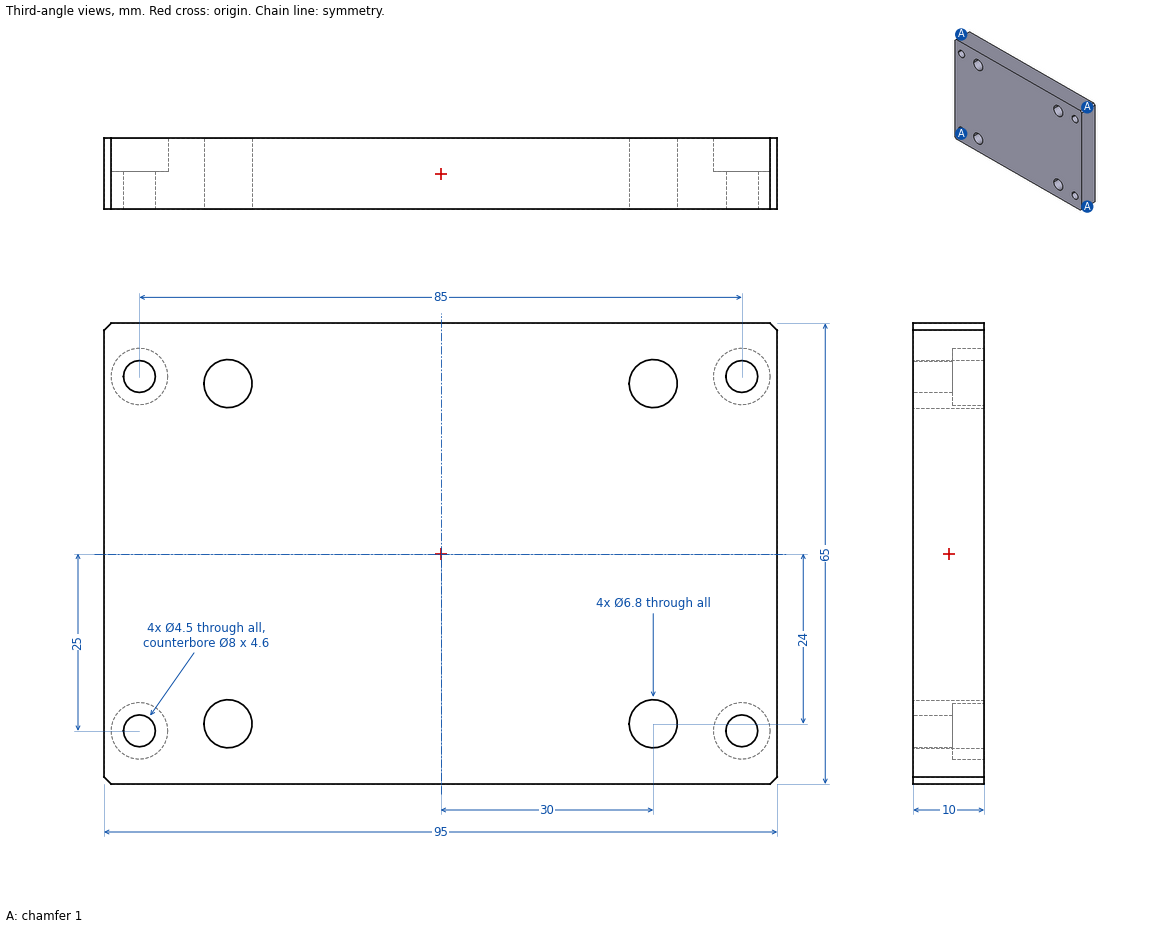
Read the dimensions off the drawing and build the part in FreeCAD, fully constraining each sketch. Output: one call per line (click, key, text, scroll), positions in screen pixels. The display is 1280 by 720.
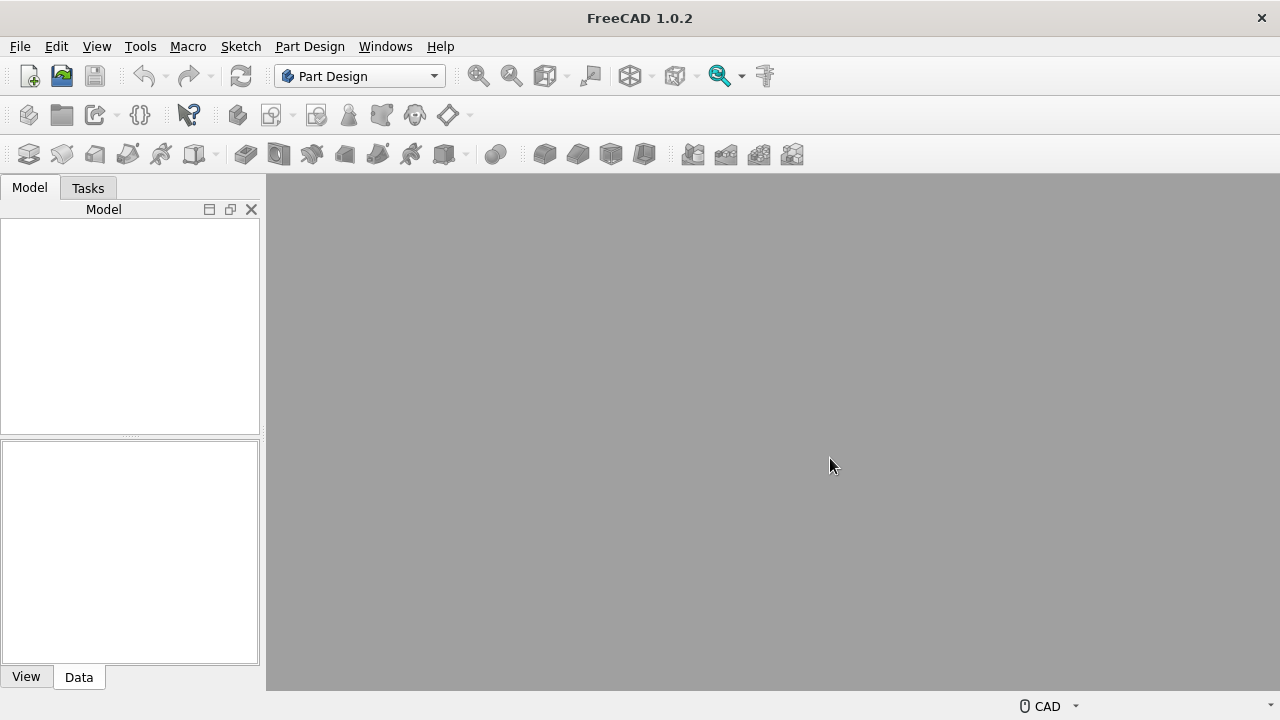
key(ctrl+n)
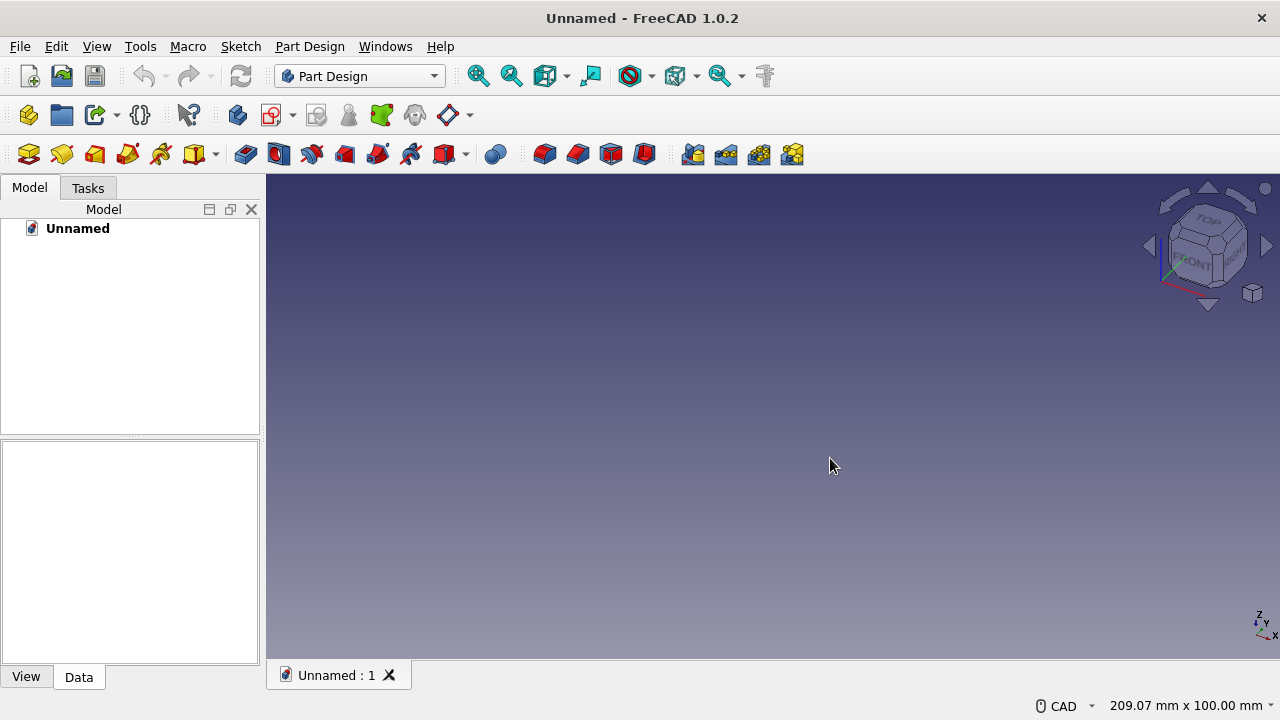
click(270, 116)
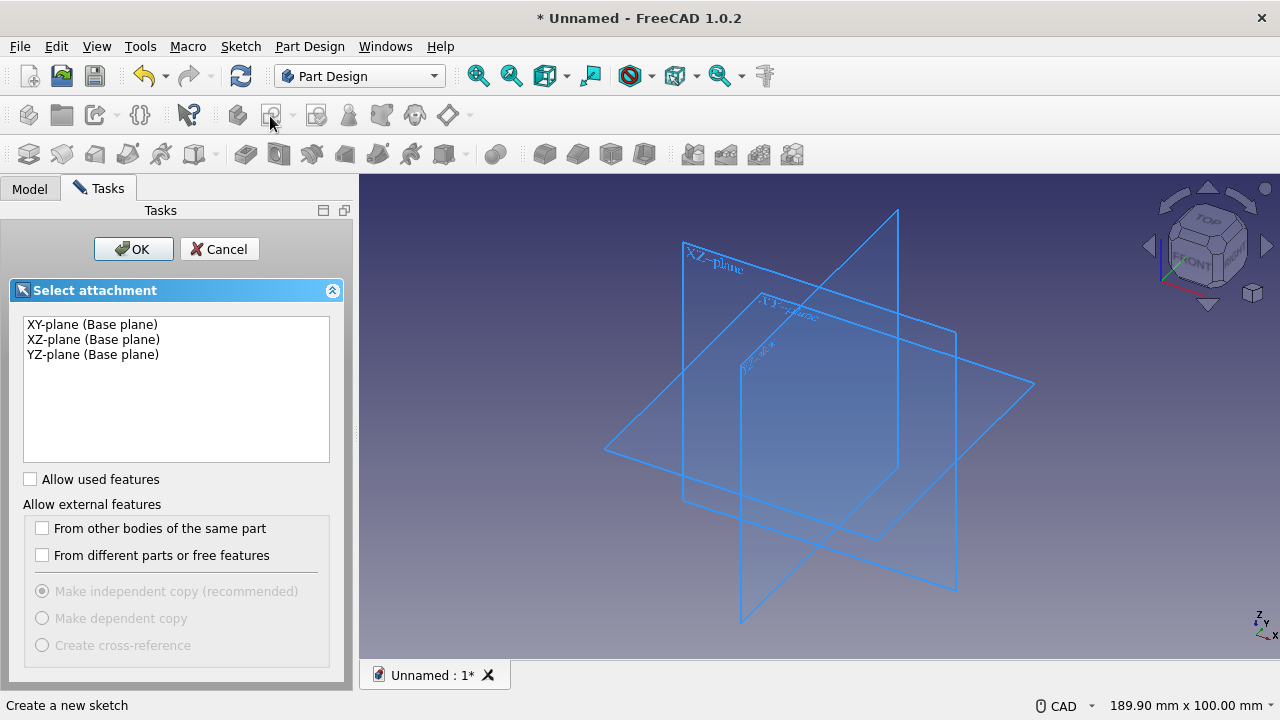
click(84, 340)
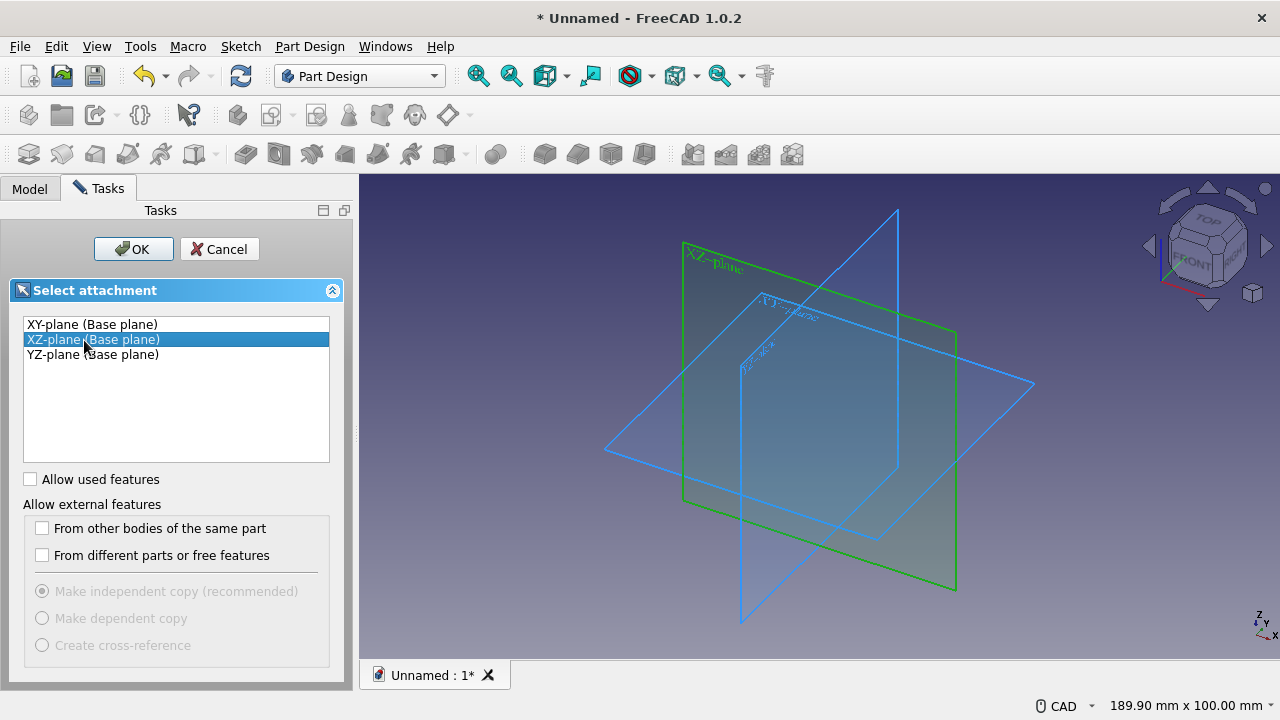
click(134, 249)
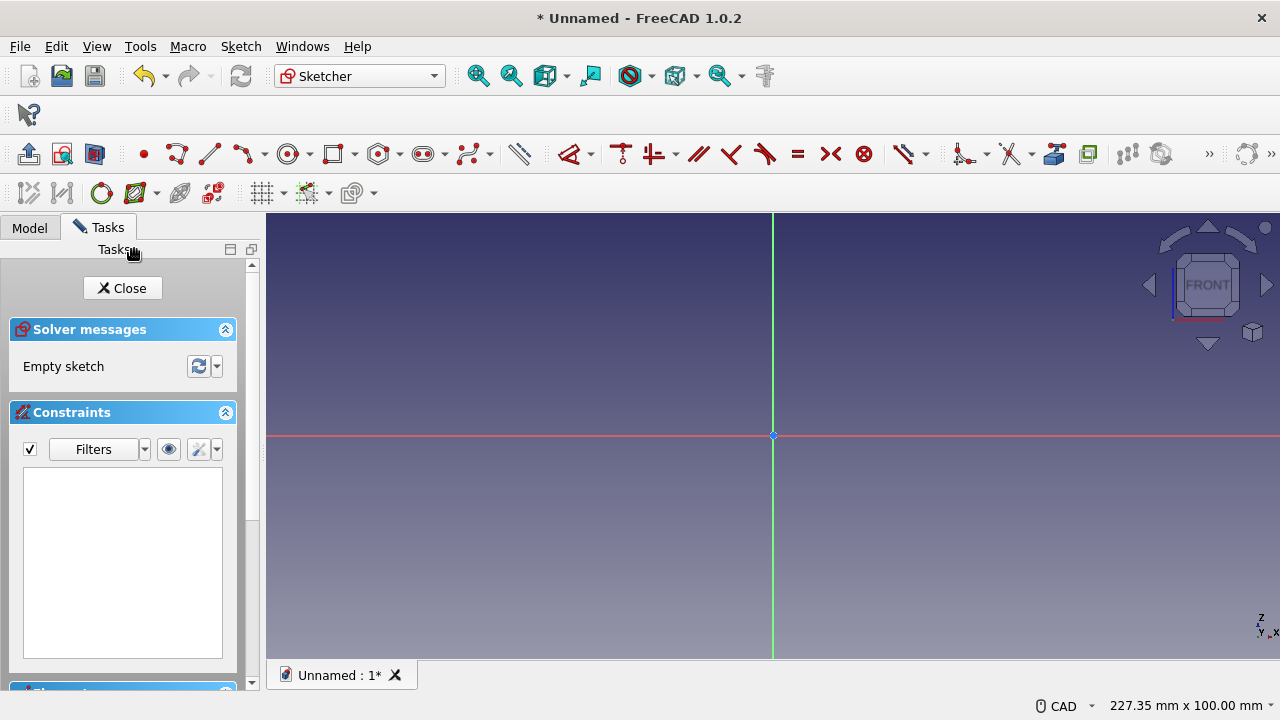
click(354, 154)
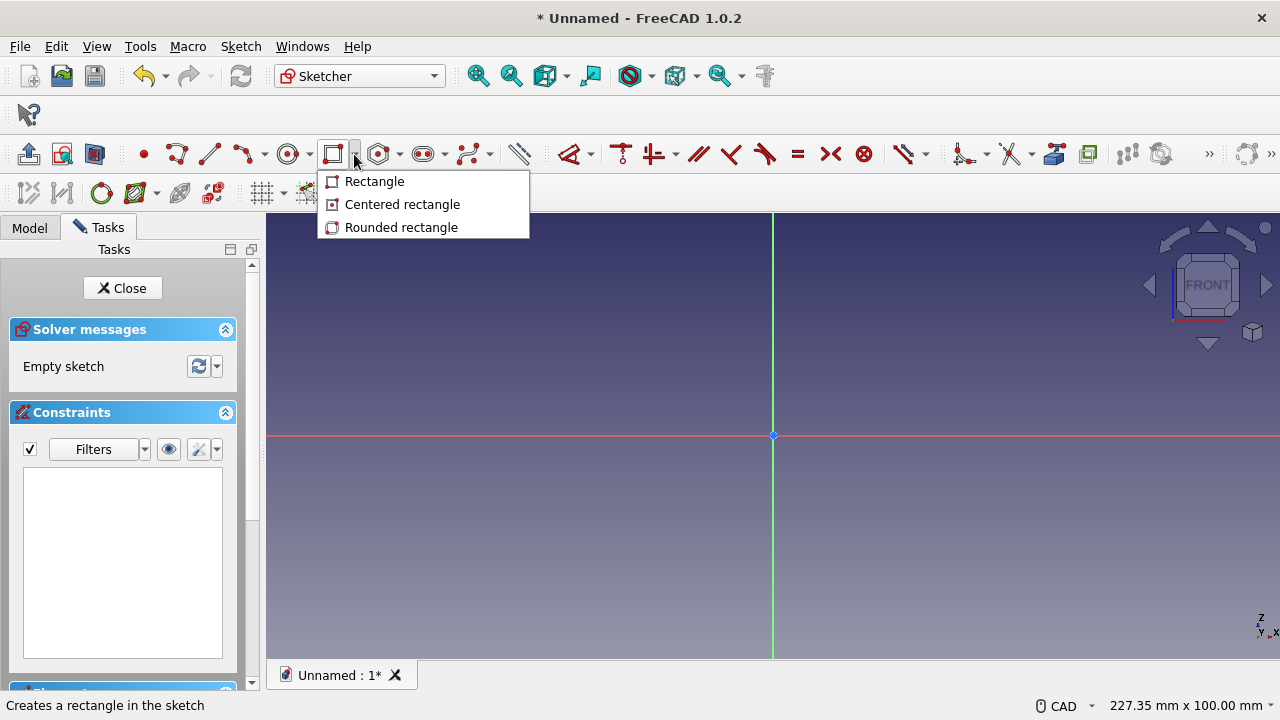
click(424, 204)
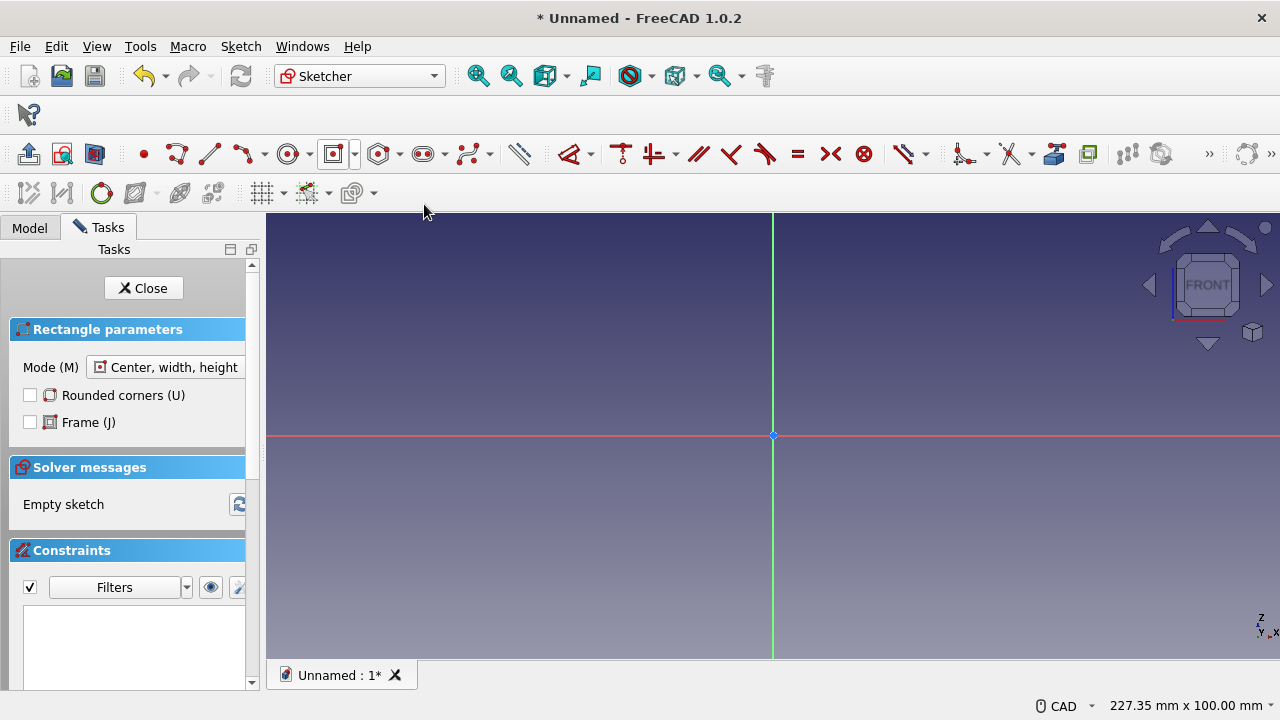
click(773, 436)
move(985, 291)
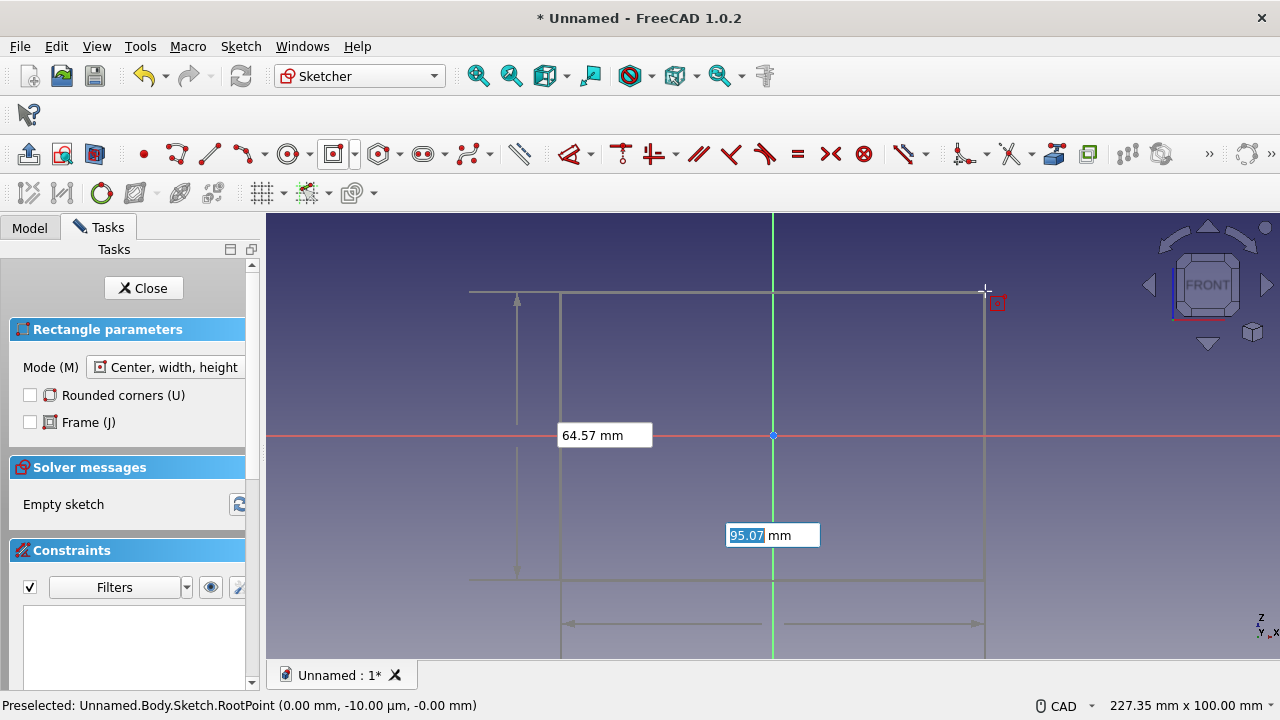
text(95)
key(Tab)
text(65)
key(Return)
key(Escape)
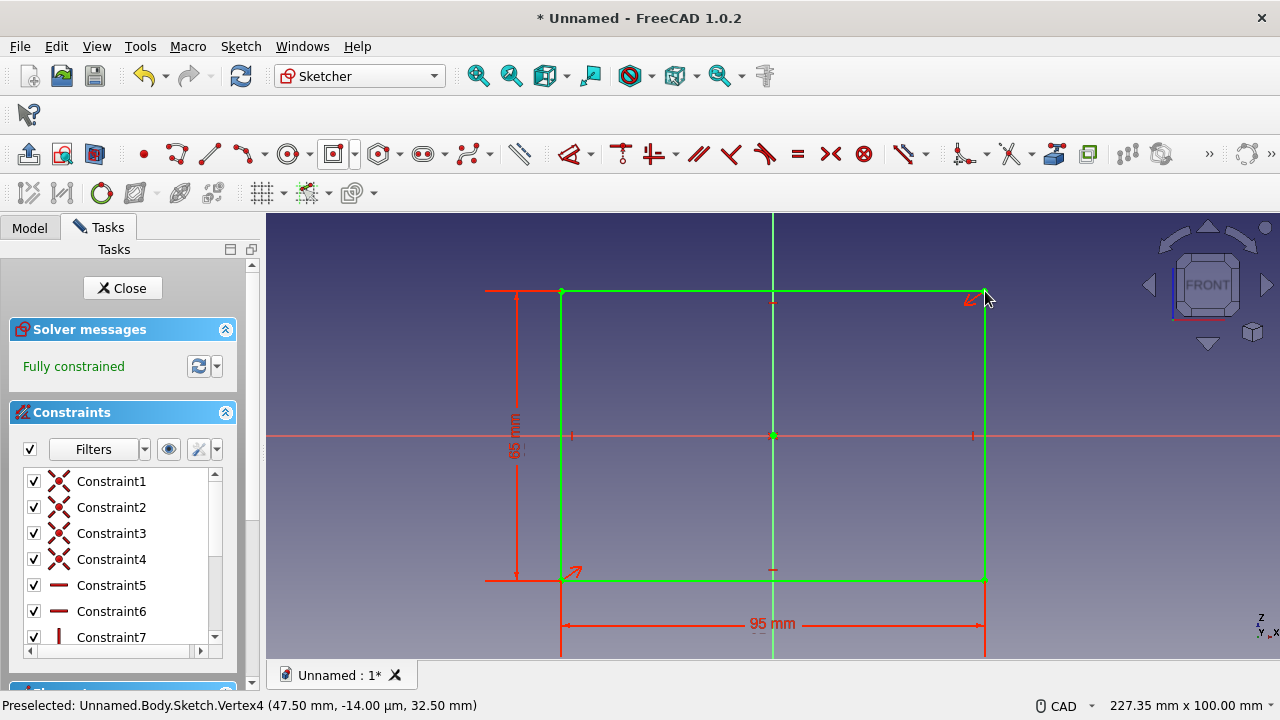
click(123, 288)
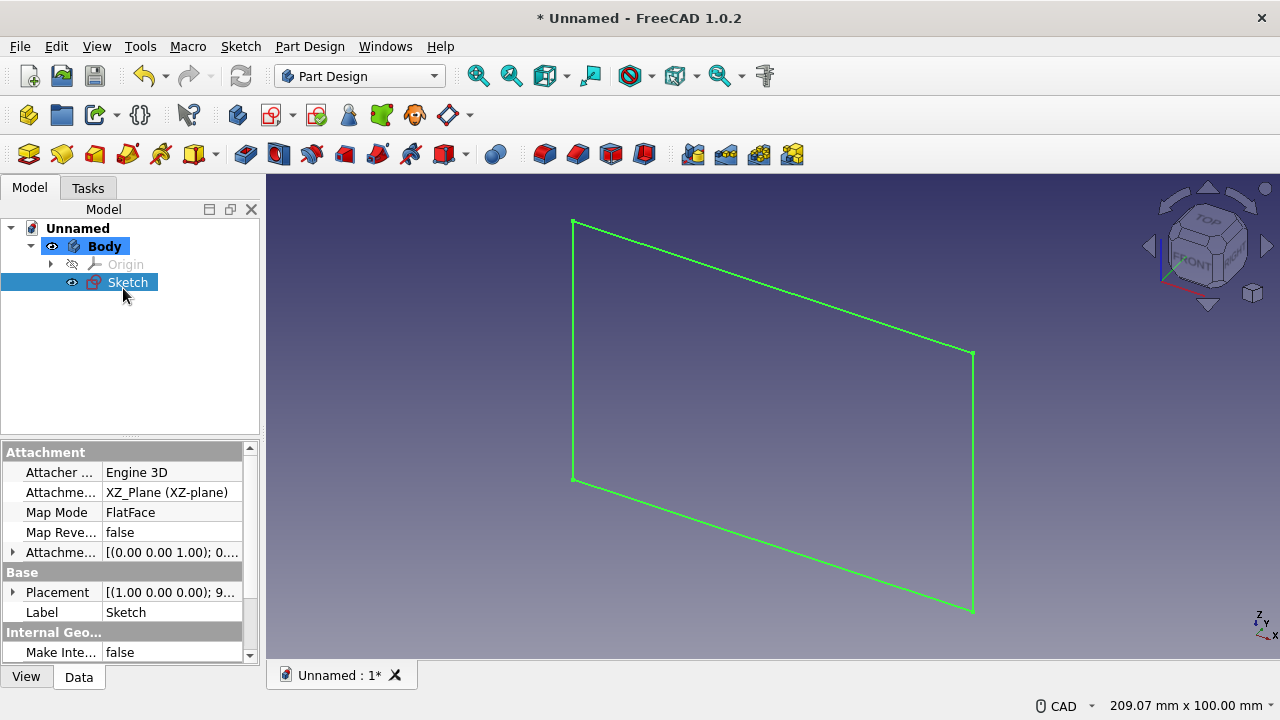
click(29, 154)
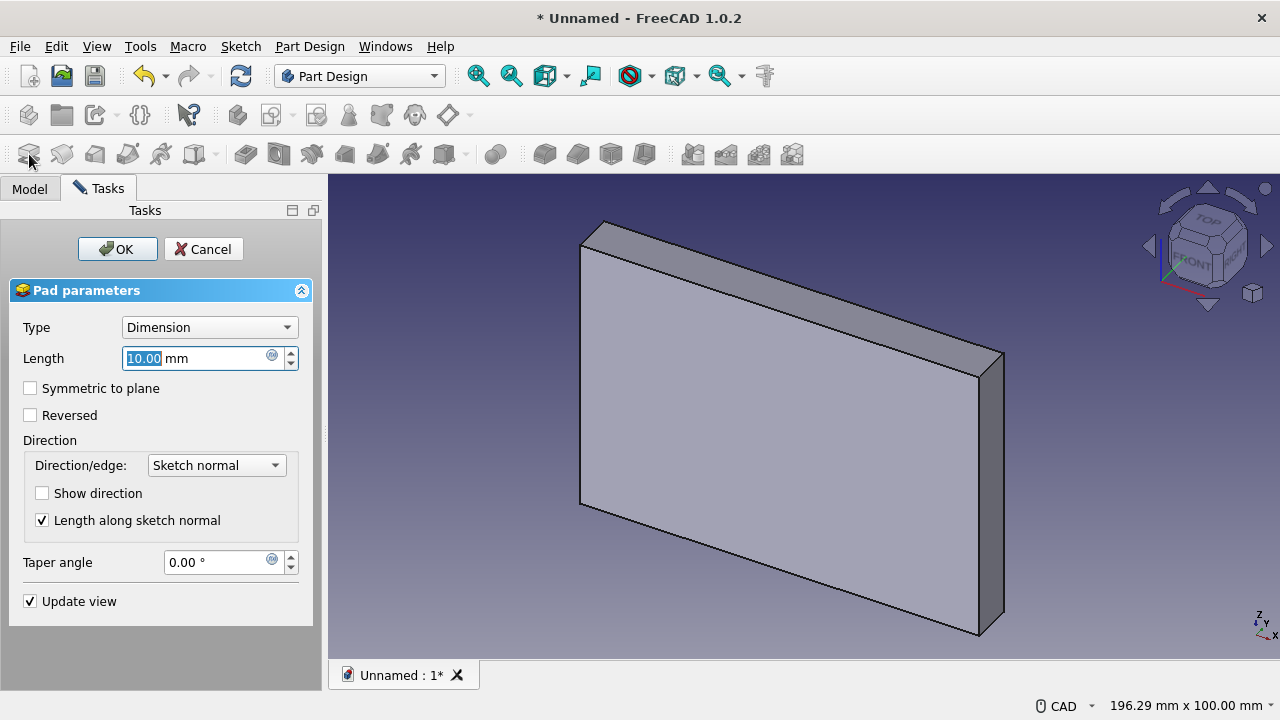
text(10)
key(Tab)